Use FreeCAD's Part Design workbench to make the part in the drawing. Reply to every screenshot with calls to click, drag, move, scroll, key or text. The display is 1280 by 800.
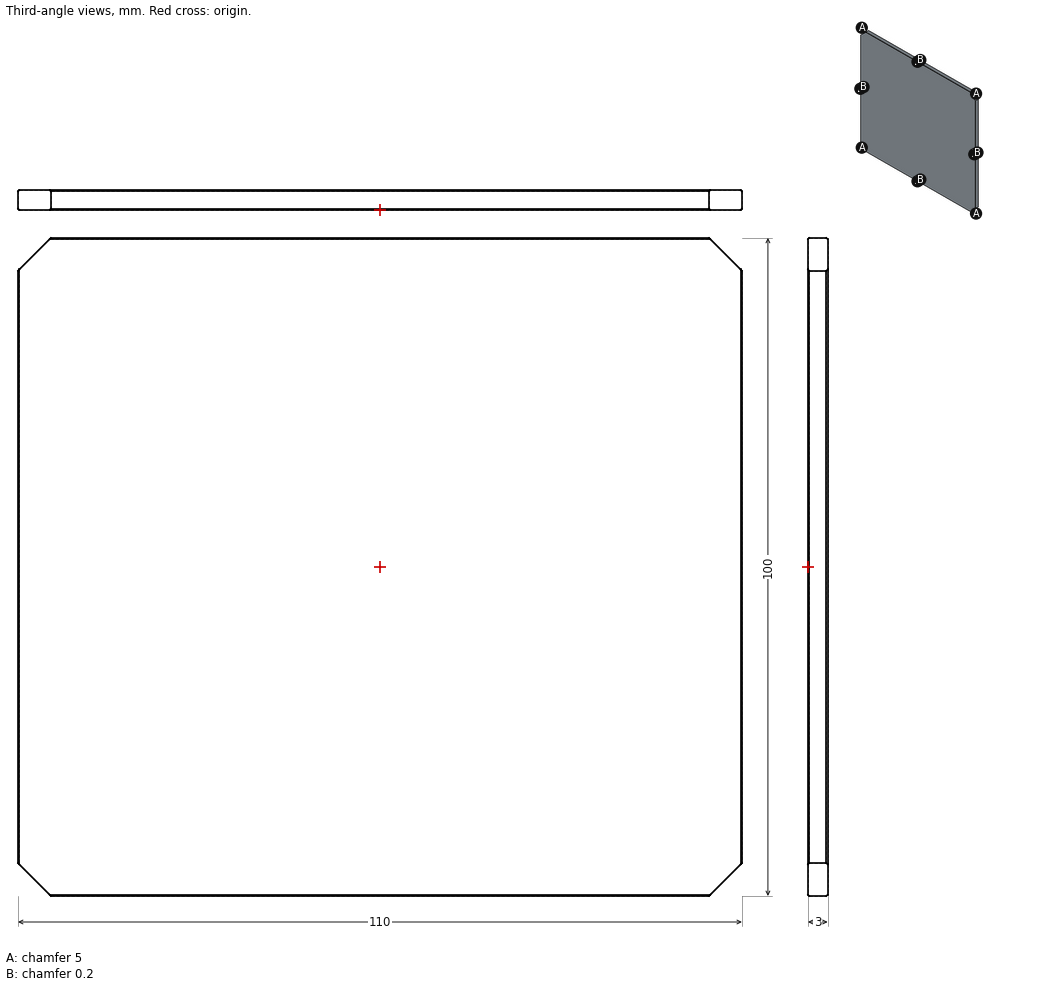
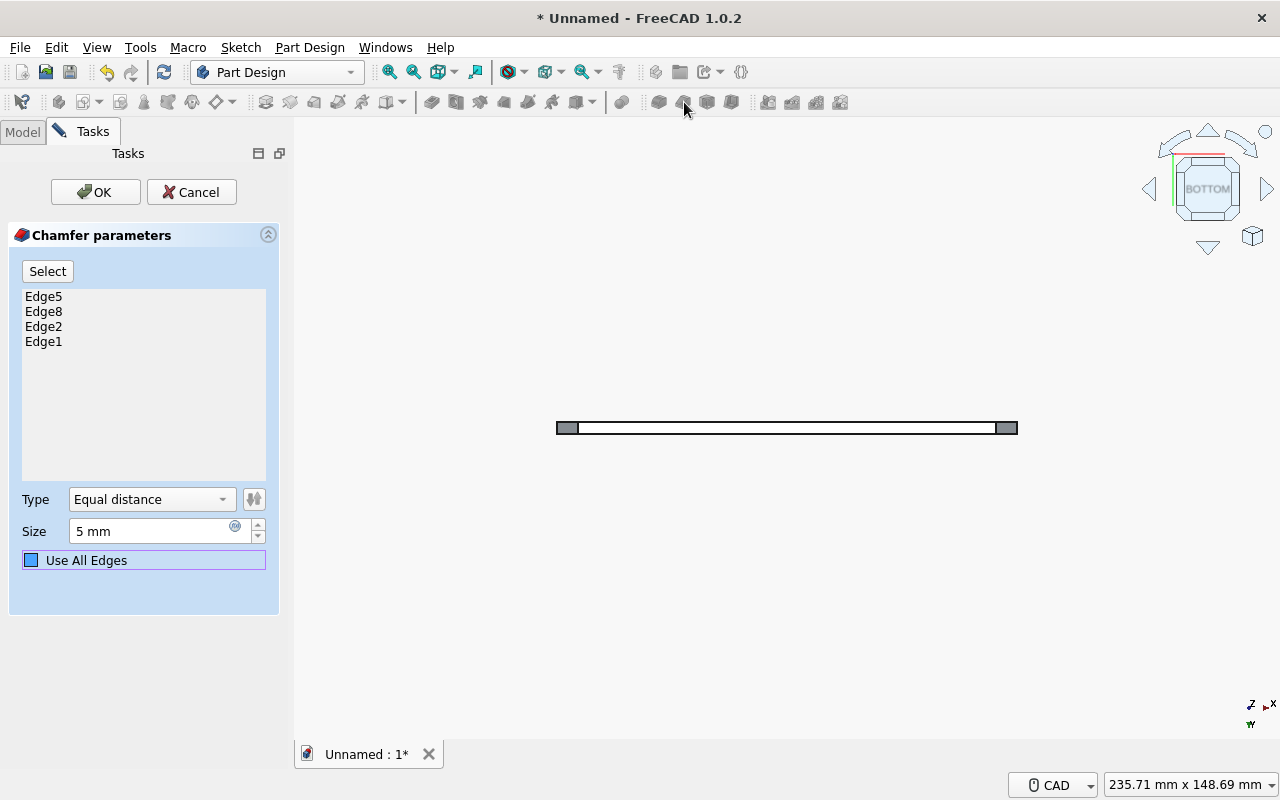
click(96, 192)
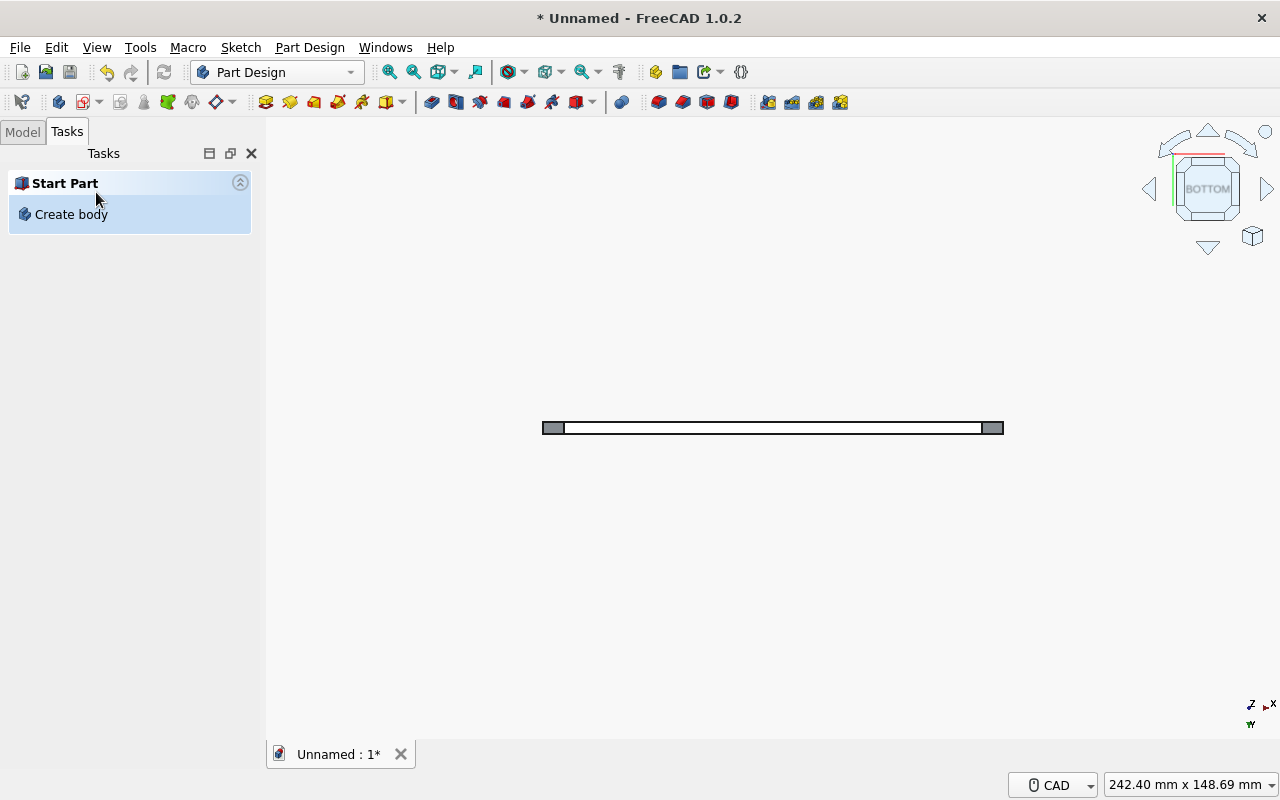
click(773, 421)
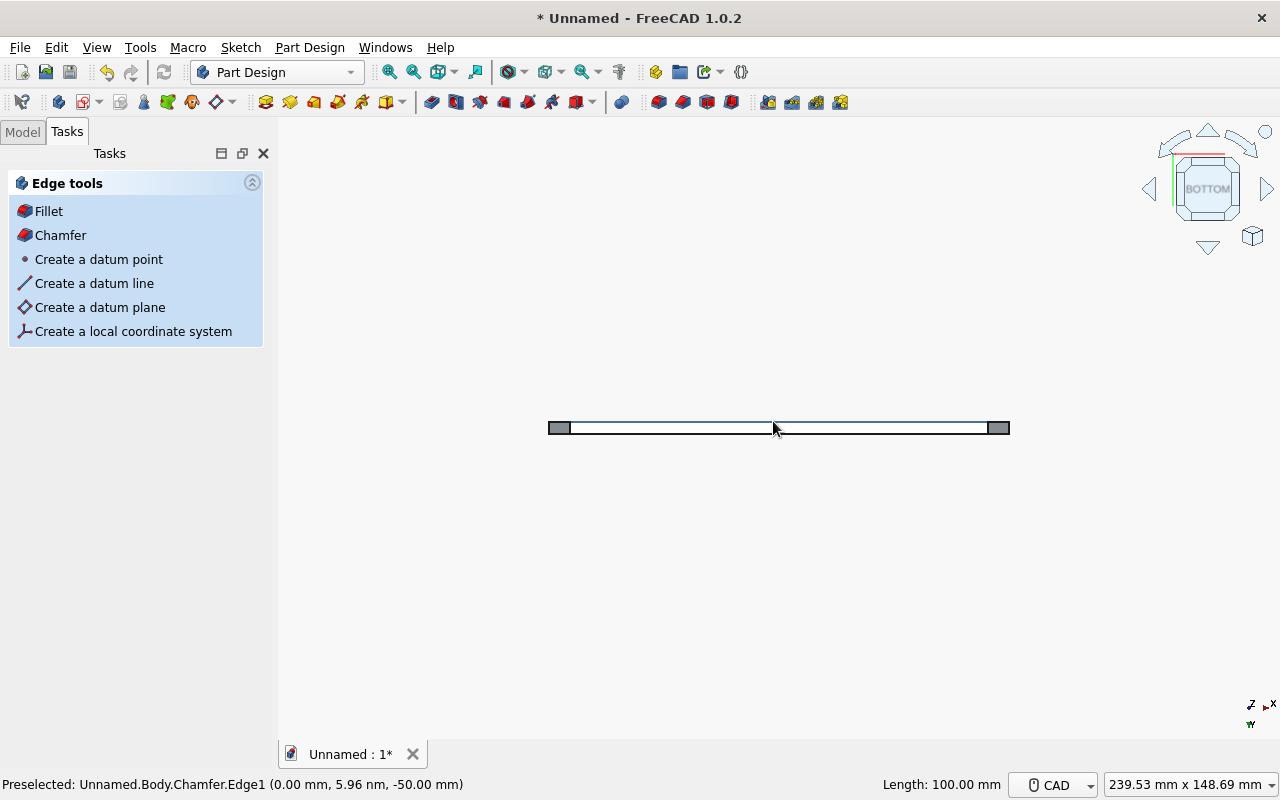
key(0)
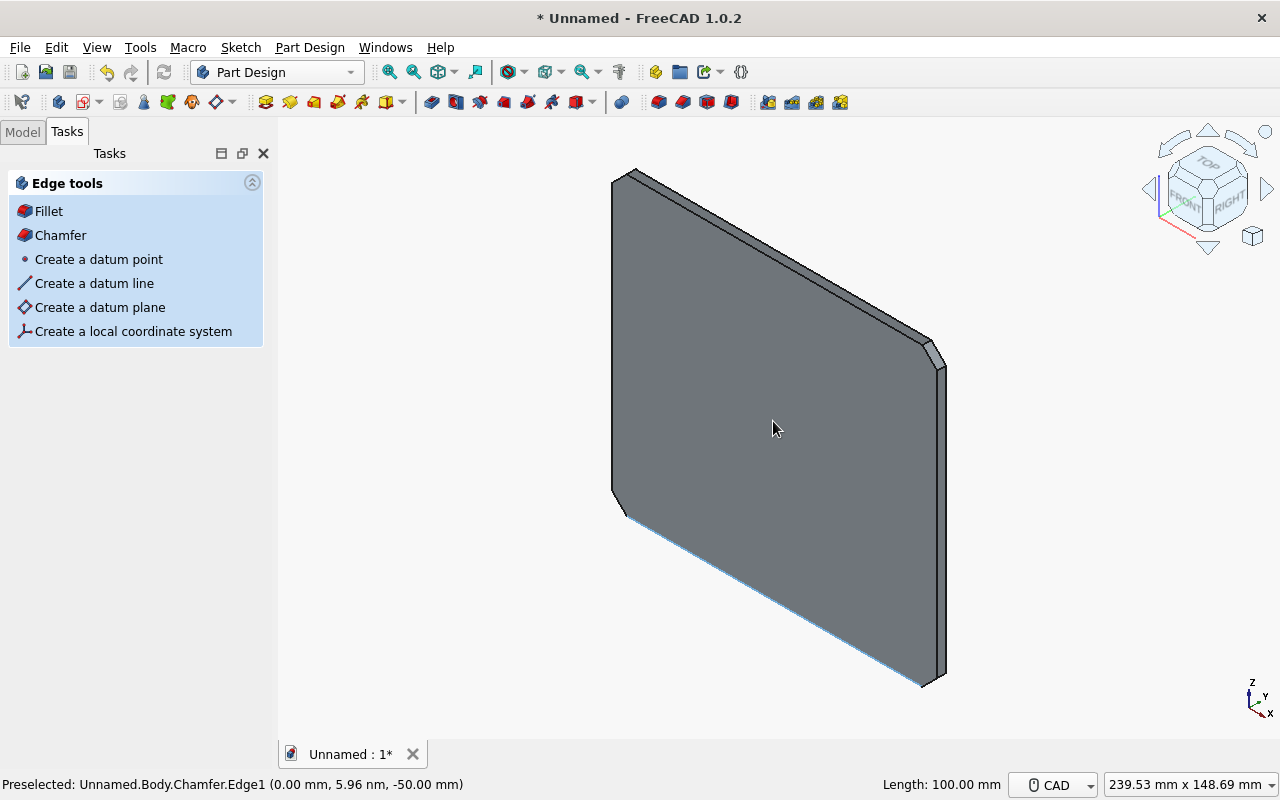
click(775, 259, ctrl)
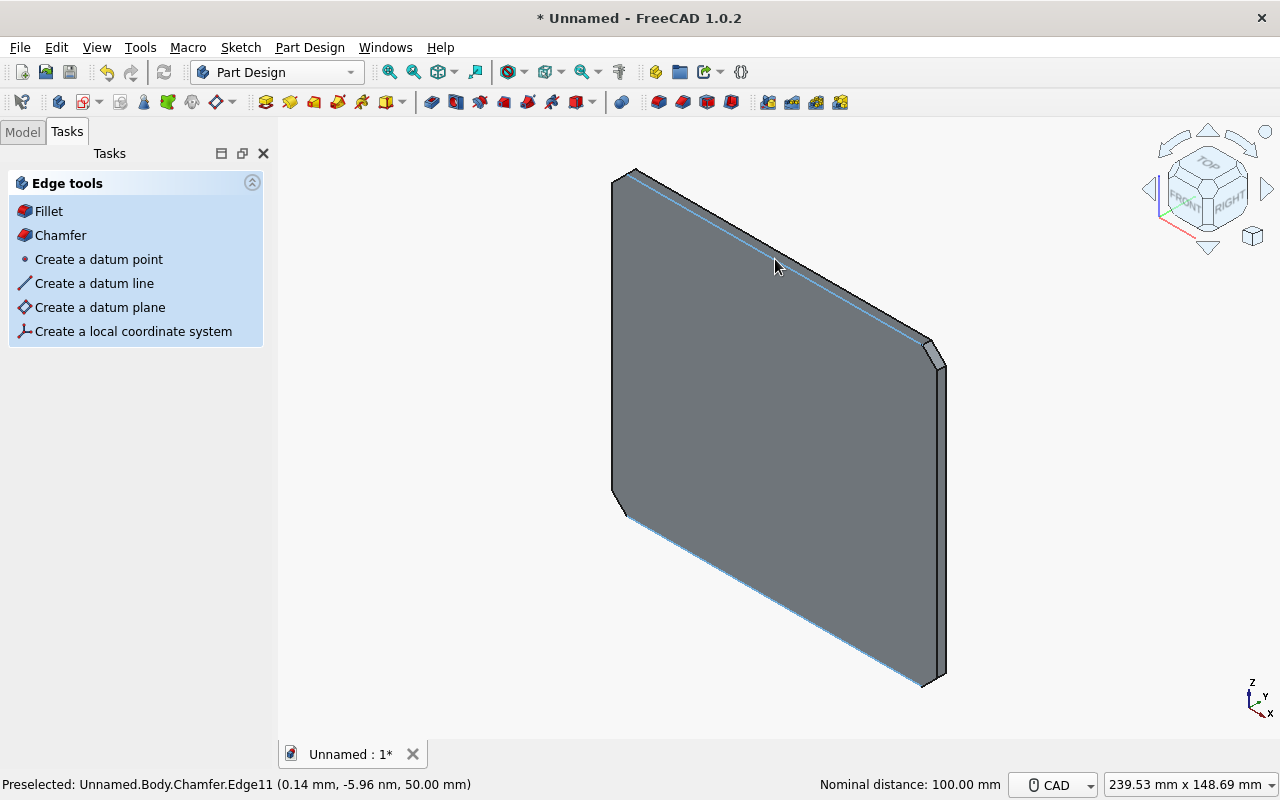
click(937, 523, ctrl)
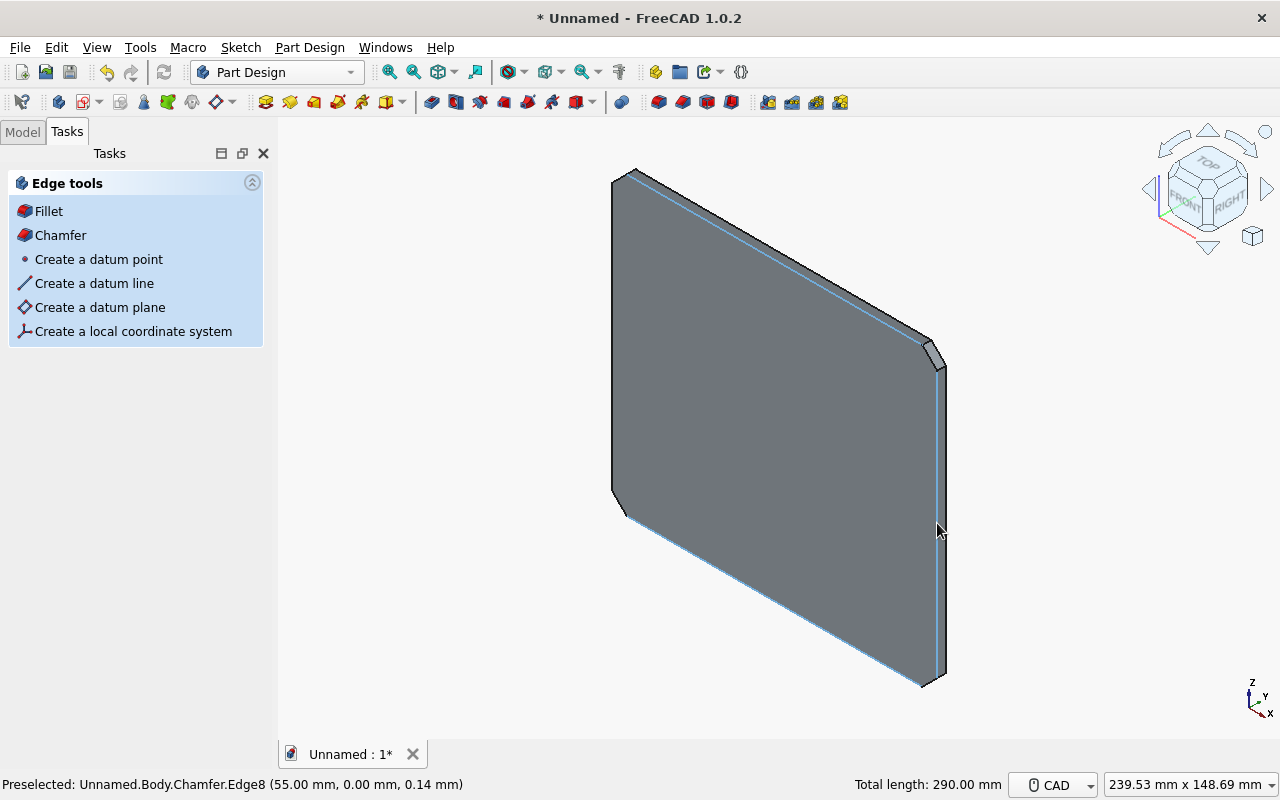
key(2)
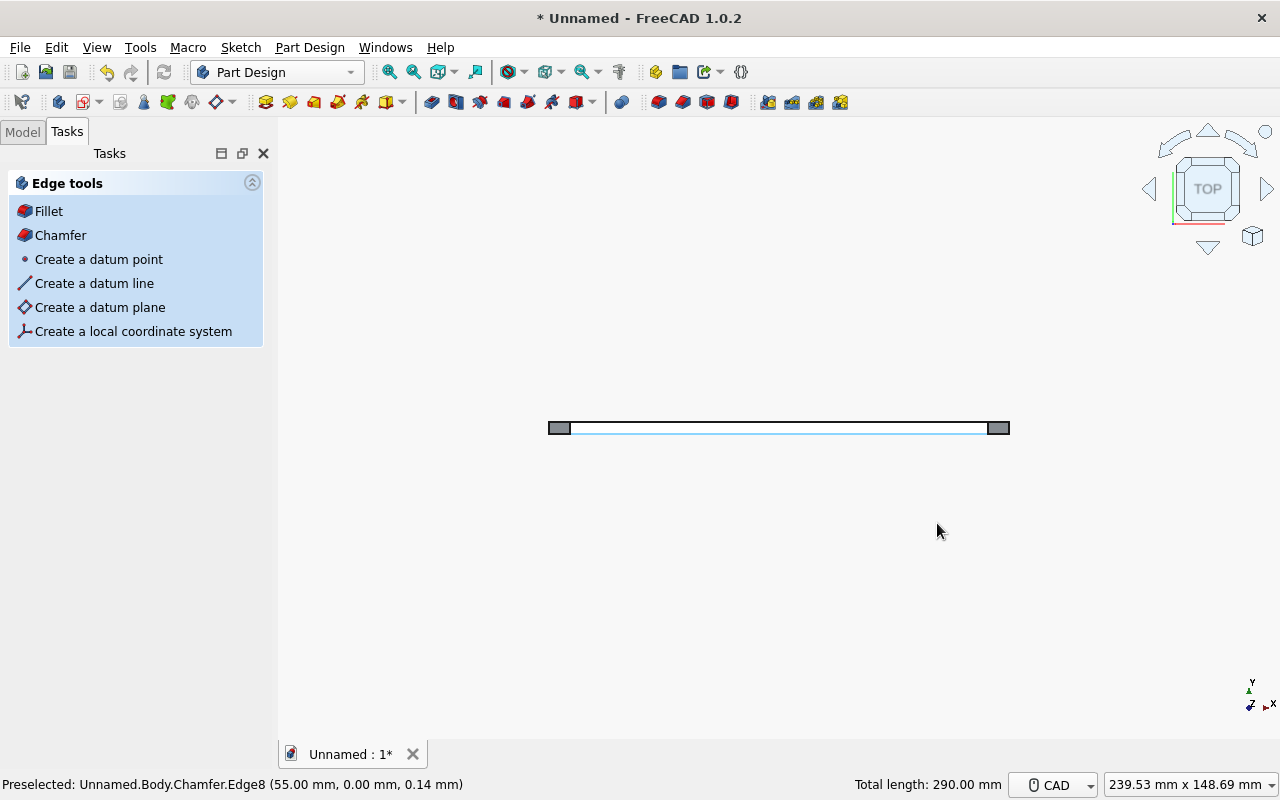
click(779, 421, ctrl)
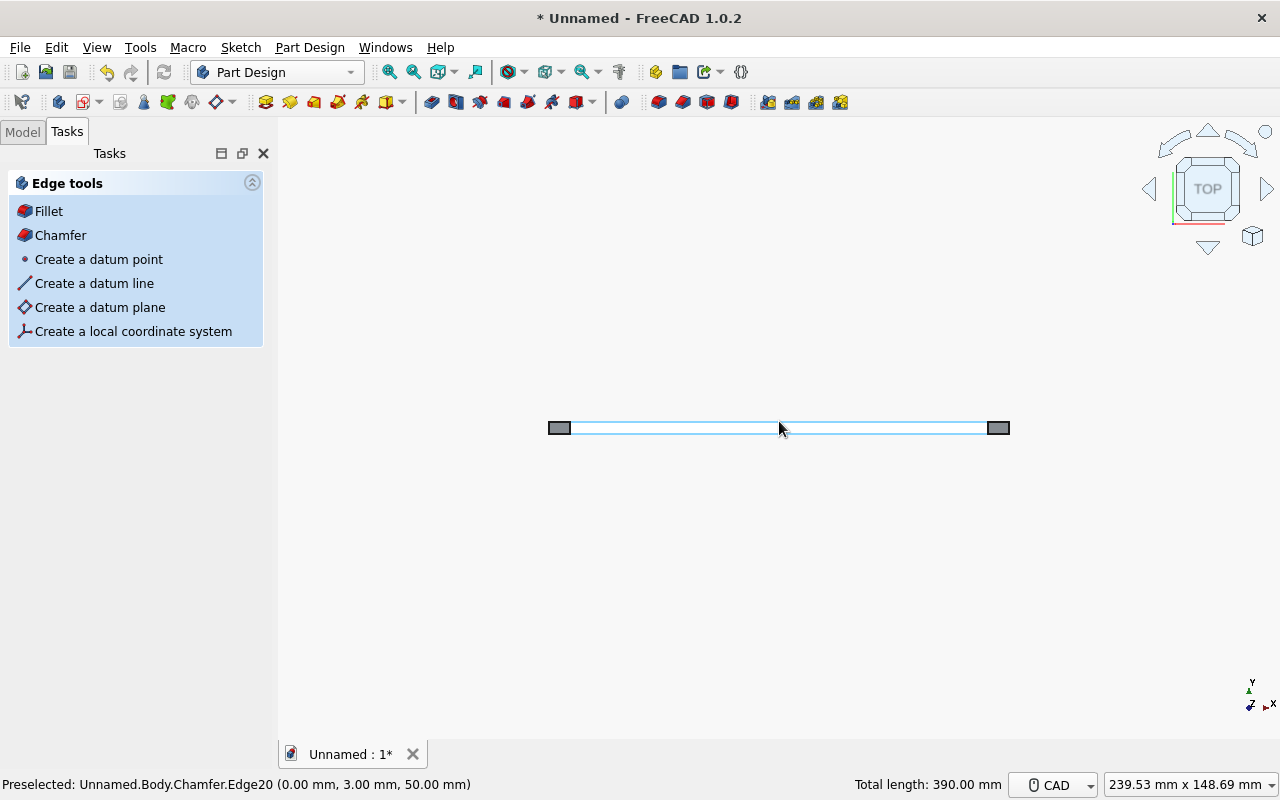
key(1)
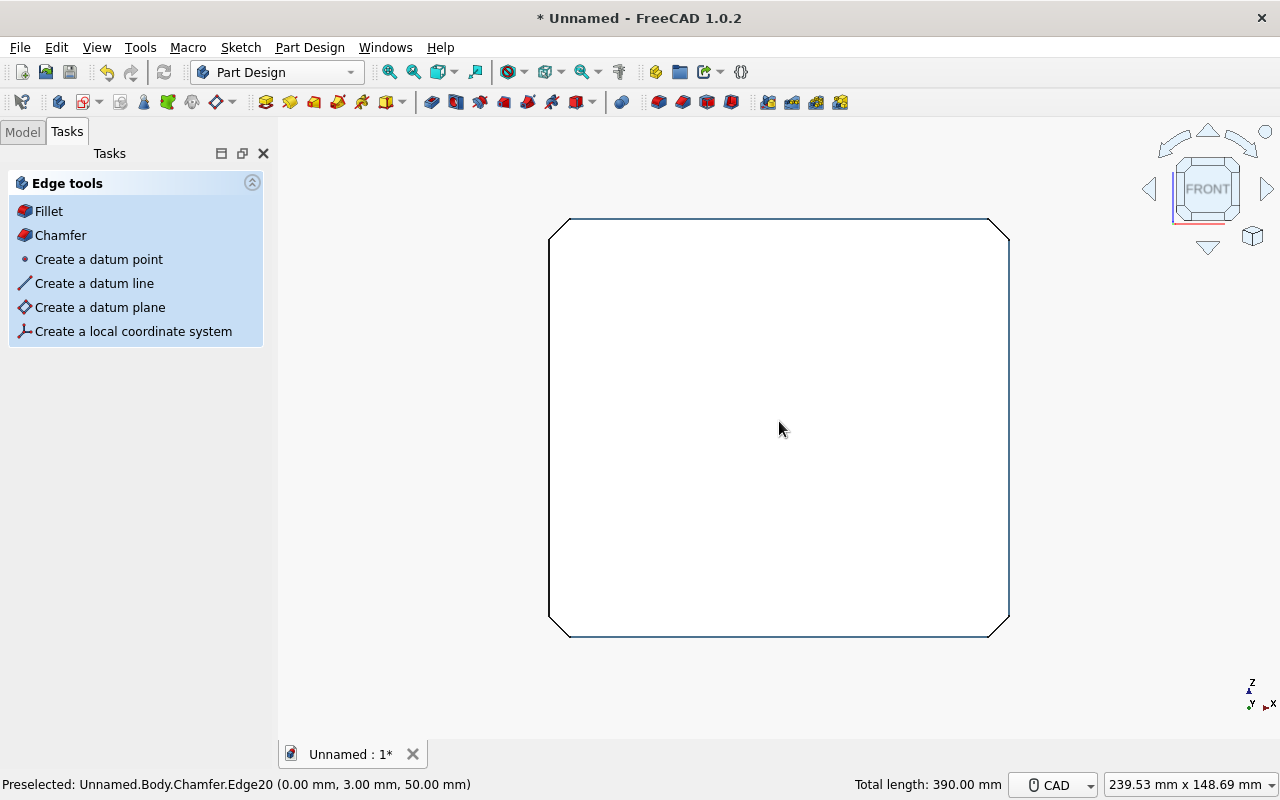
click(549, 465, ctrl)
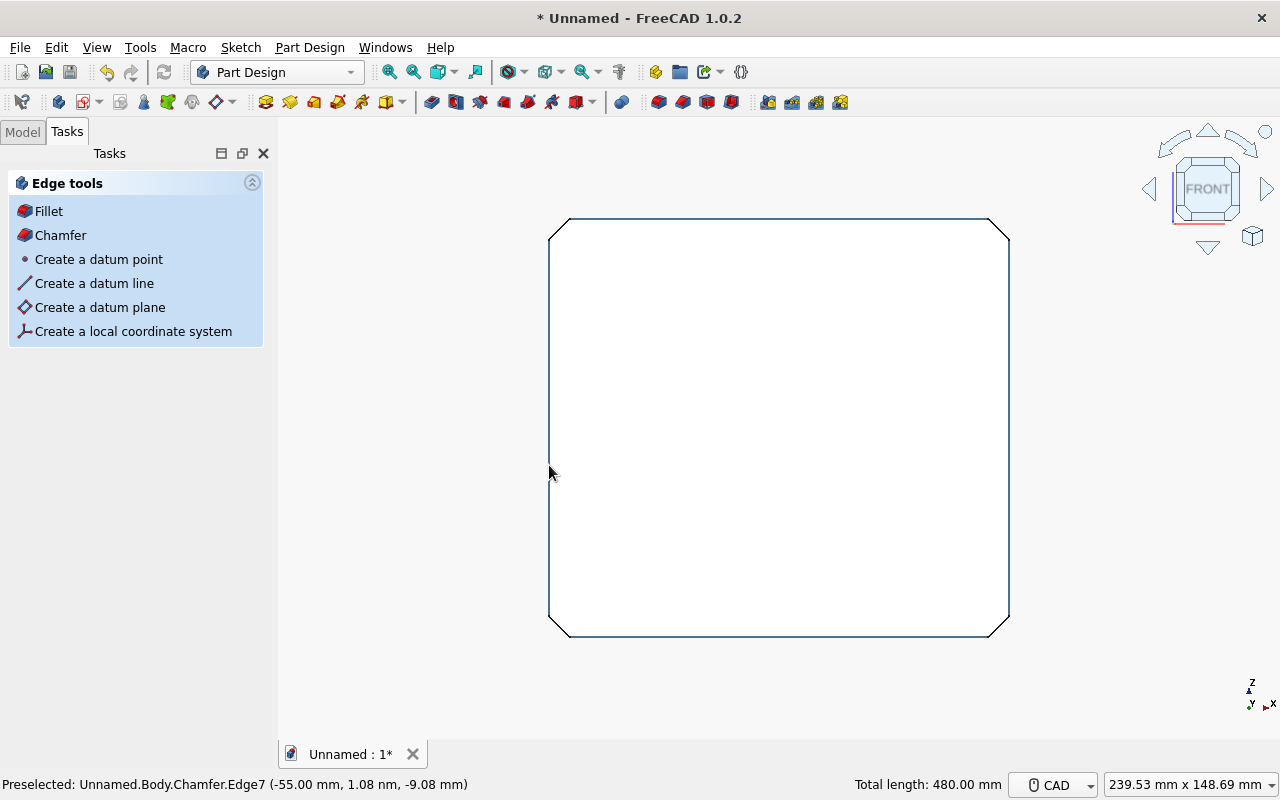
key(3)